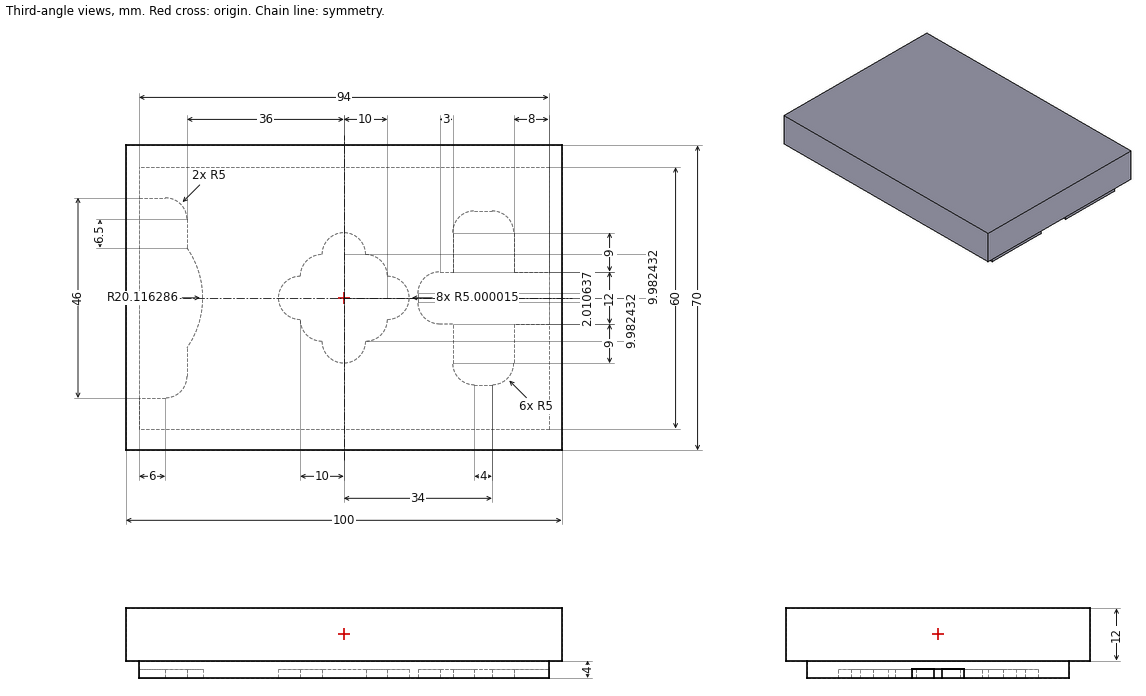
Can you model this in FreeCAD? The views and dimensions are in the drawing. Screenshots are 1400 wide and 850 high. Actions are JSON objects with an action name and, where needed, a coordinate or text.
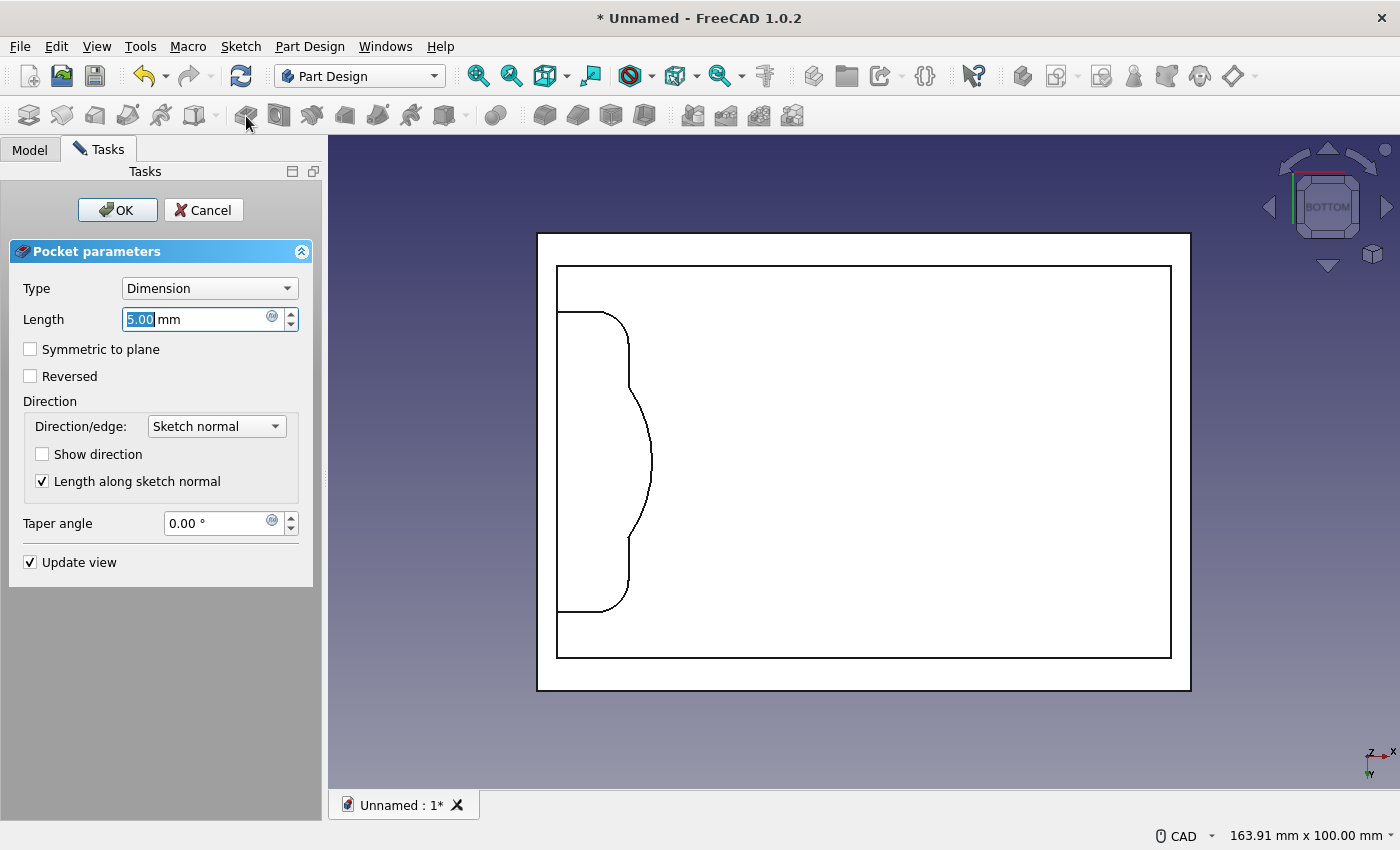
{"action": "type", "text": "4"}
{"action": "key", "text": "Tab"}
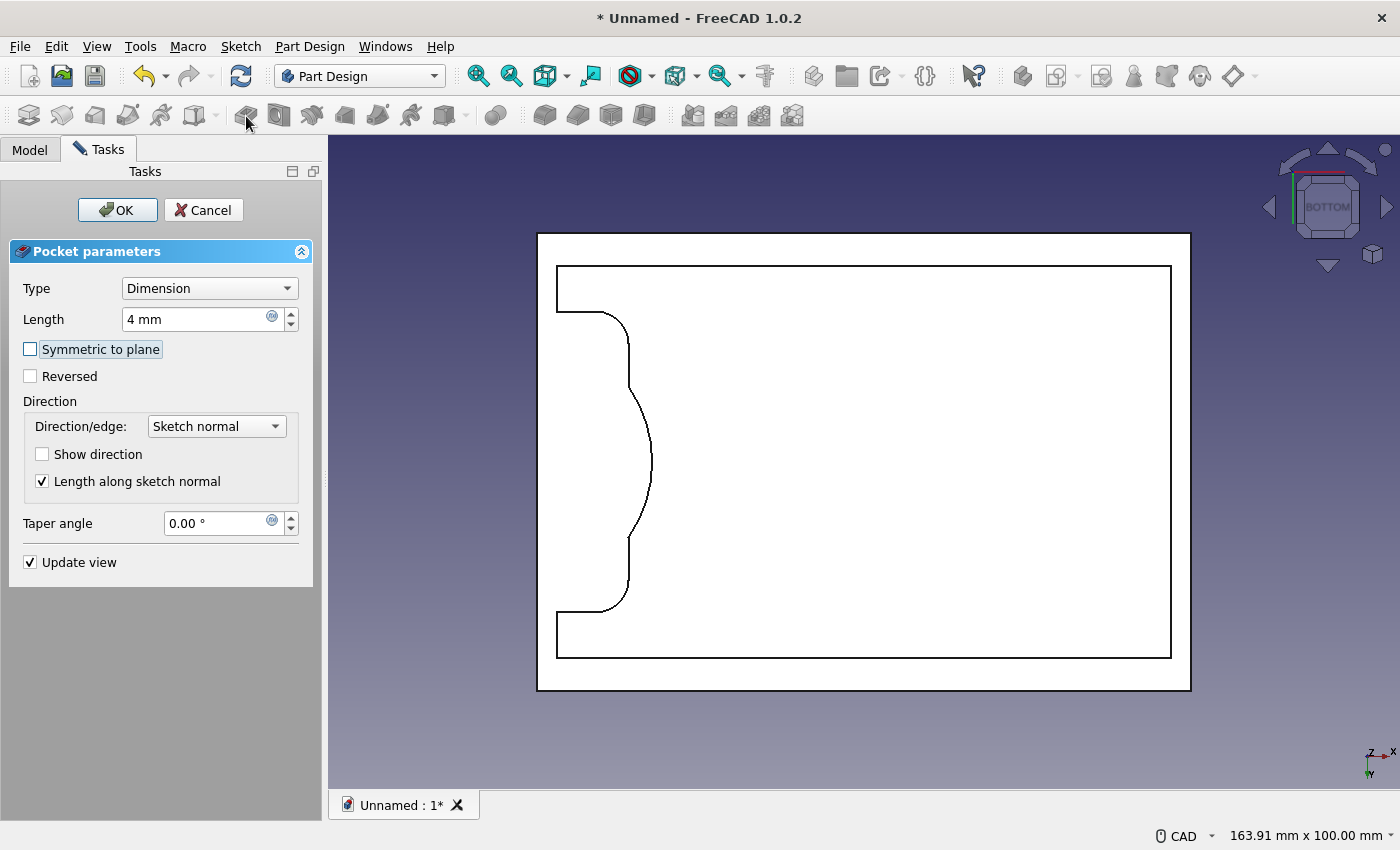
{"action": "left_click", "coordinate": [31, 349]}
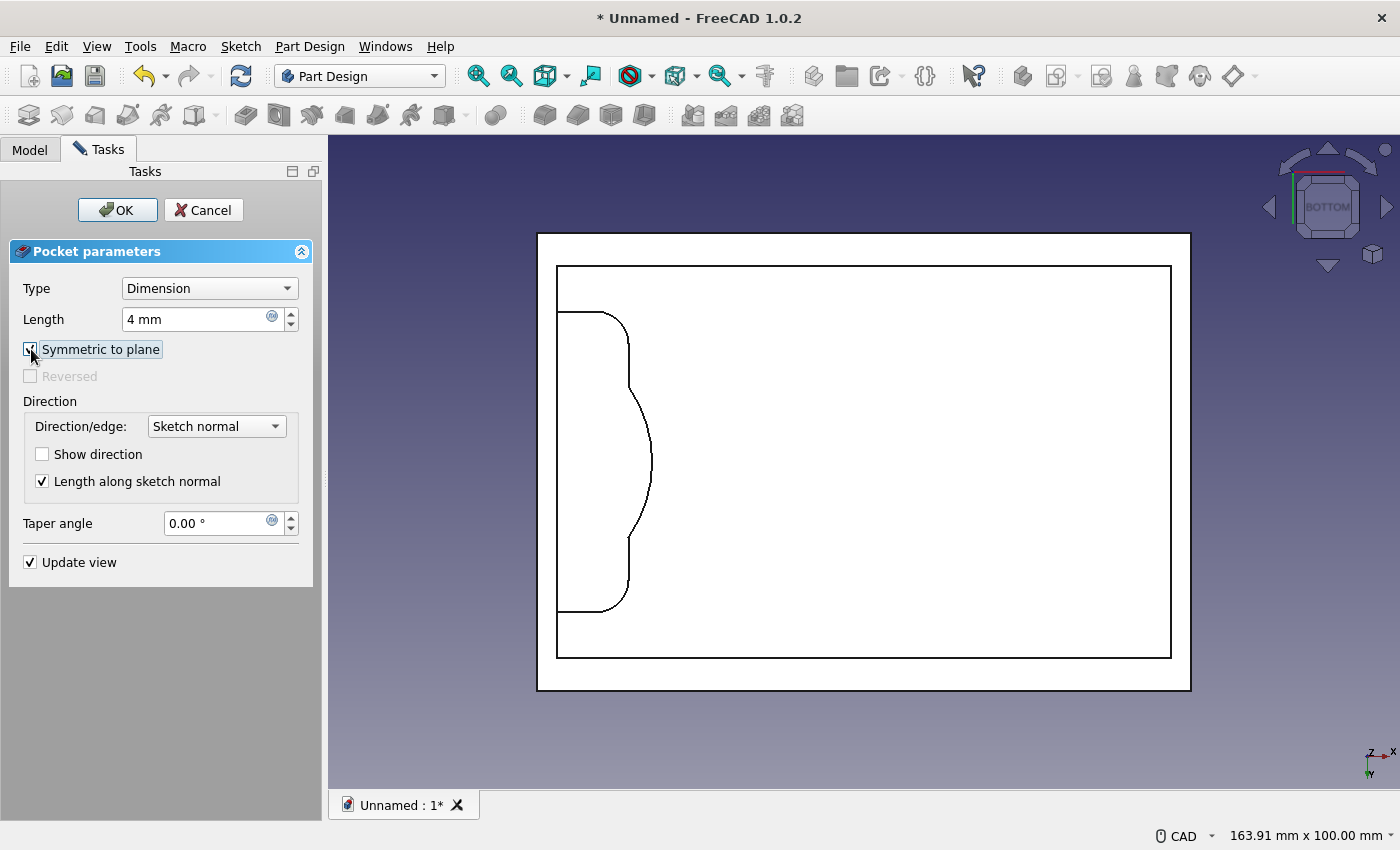
{"action": "left_click", "coordinate": [118, 210]}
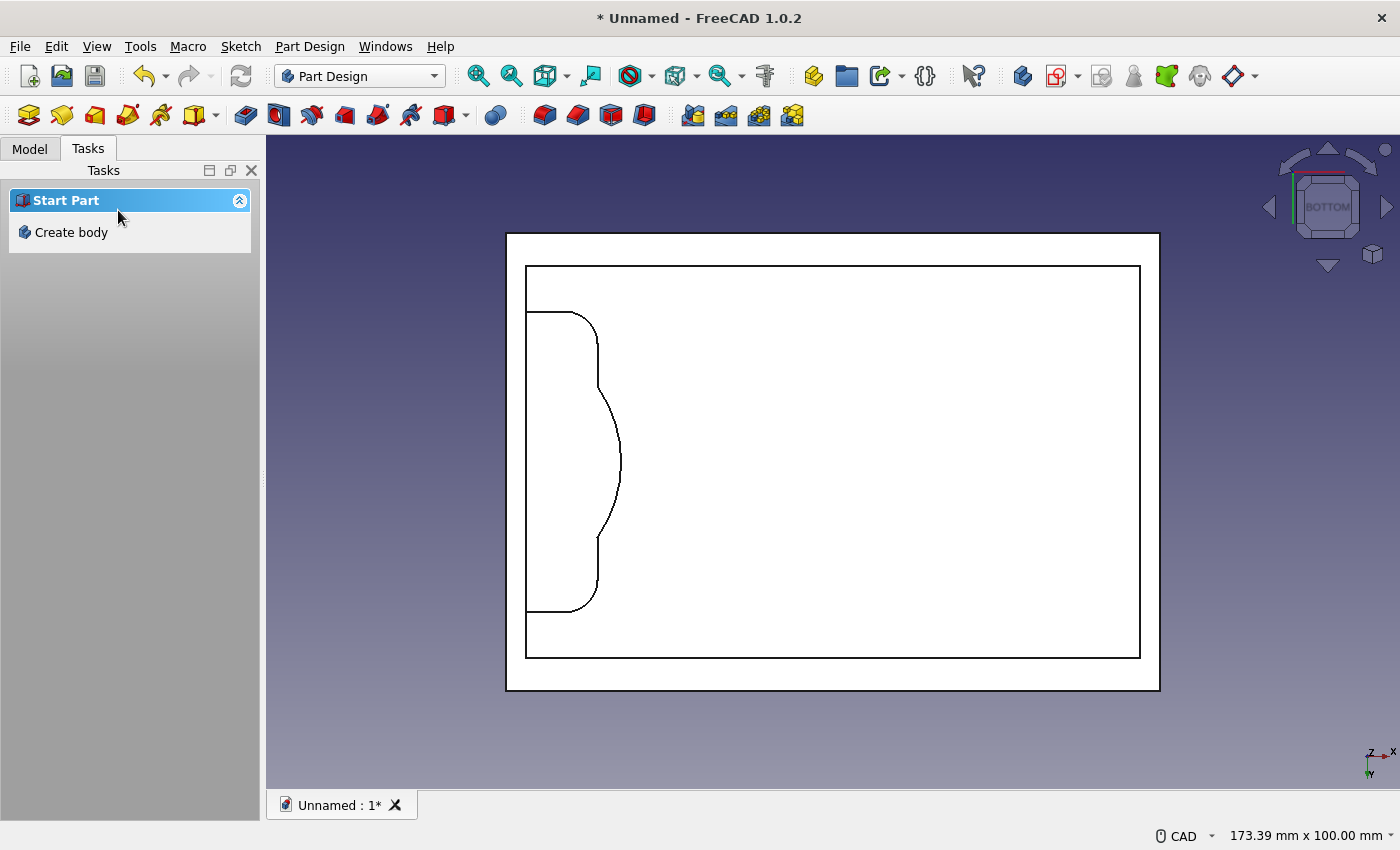
{"action": "left_click", "coordinate": [921, 461]}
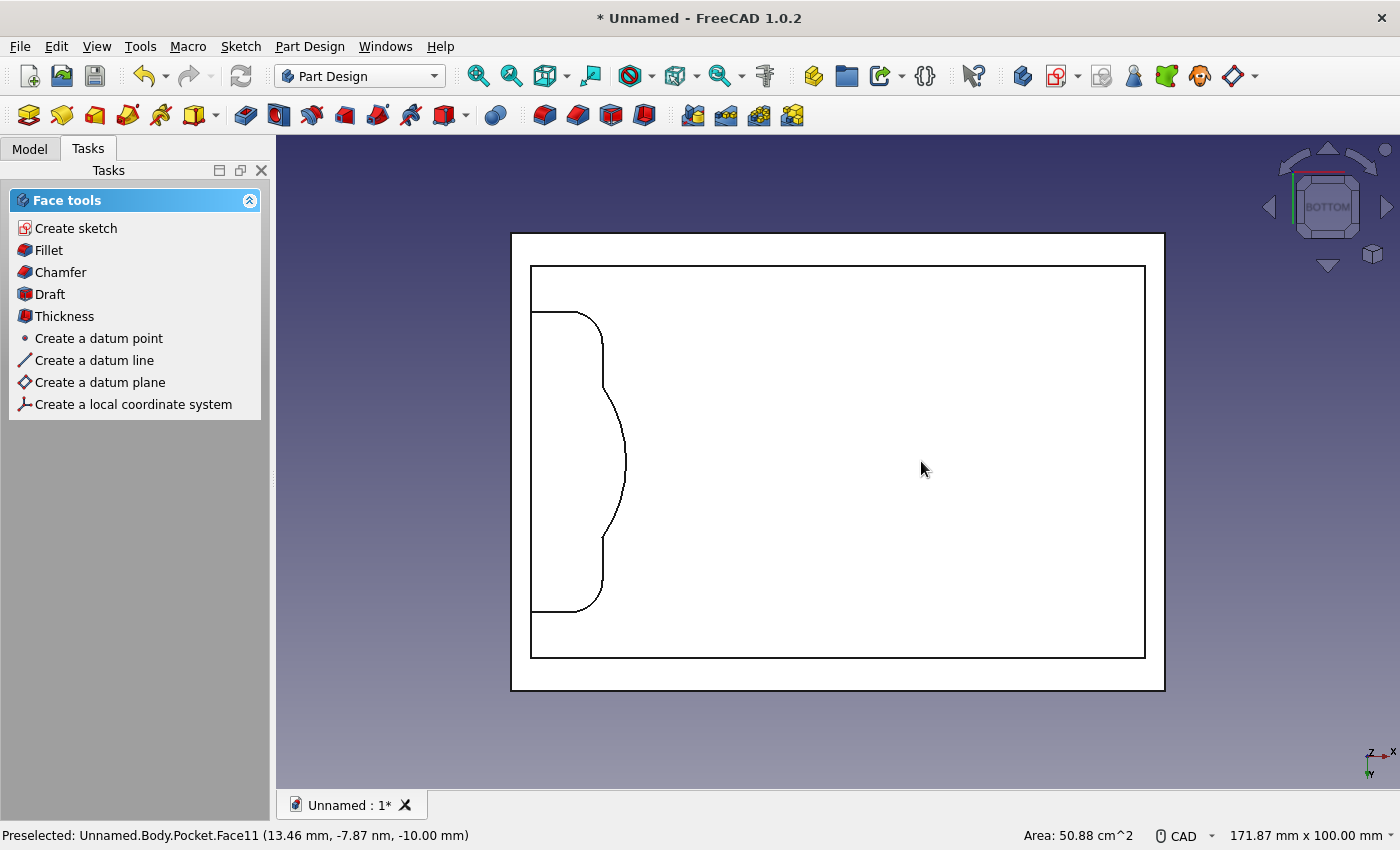
{"action": "left_click", "coordinate": [1056, 76]}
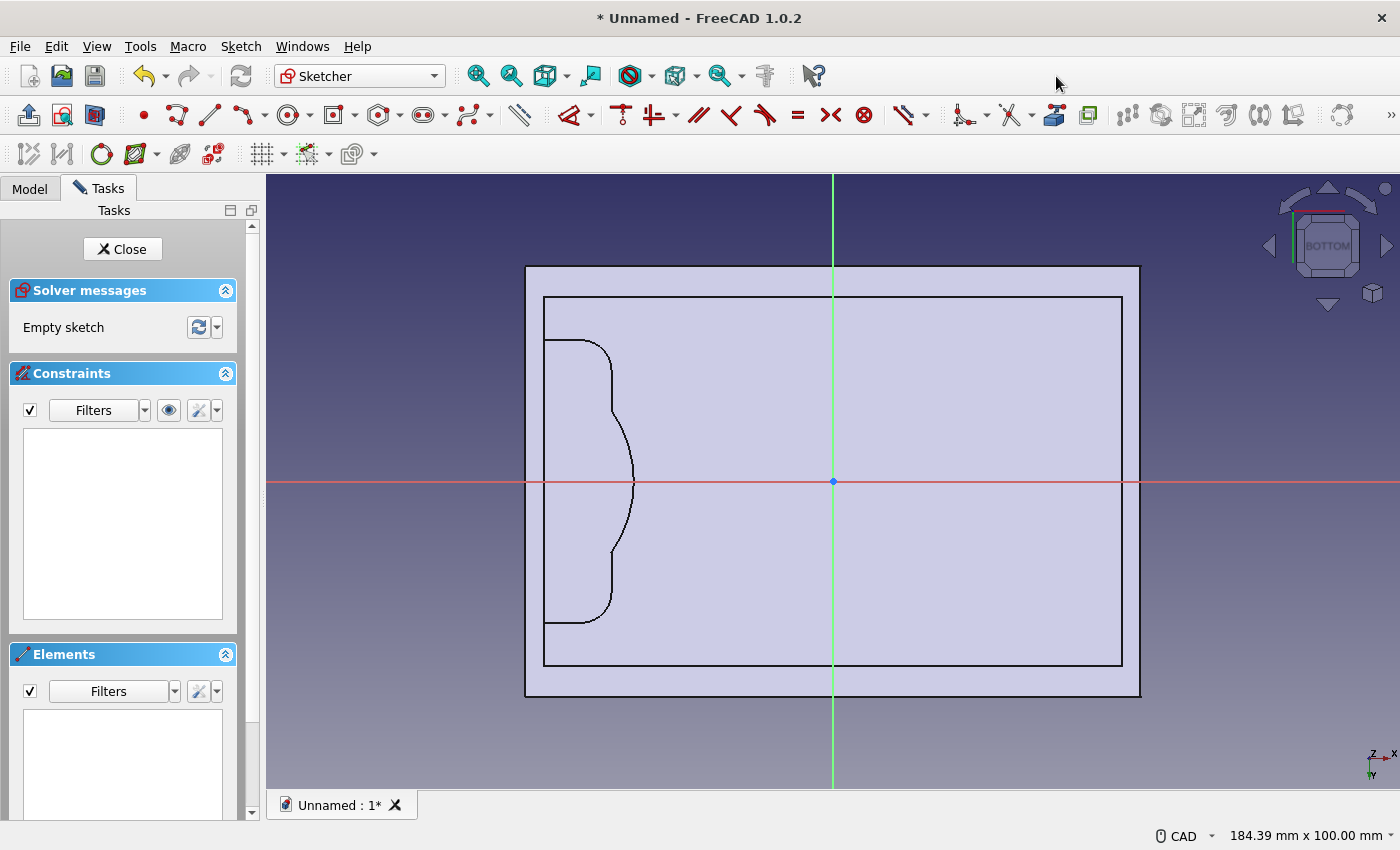
{"action": "scroll", "coordinate": [1235, 482], "scroll_direction": "up", "scroll_amount": 2}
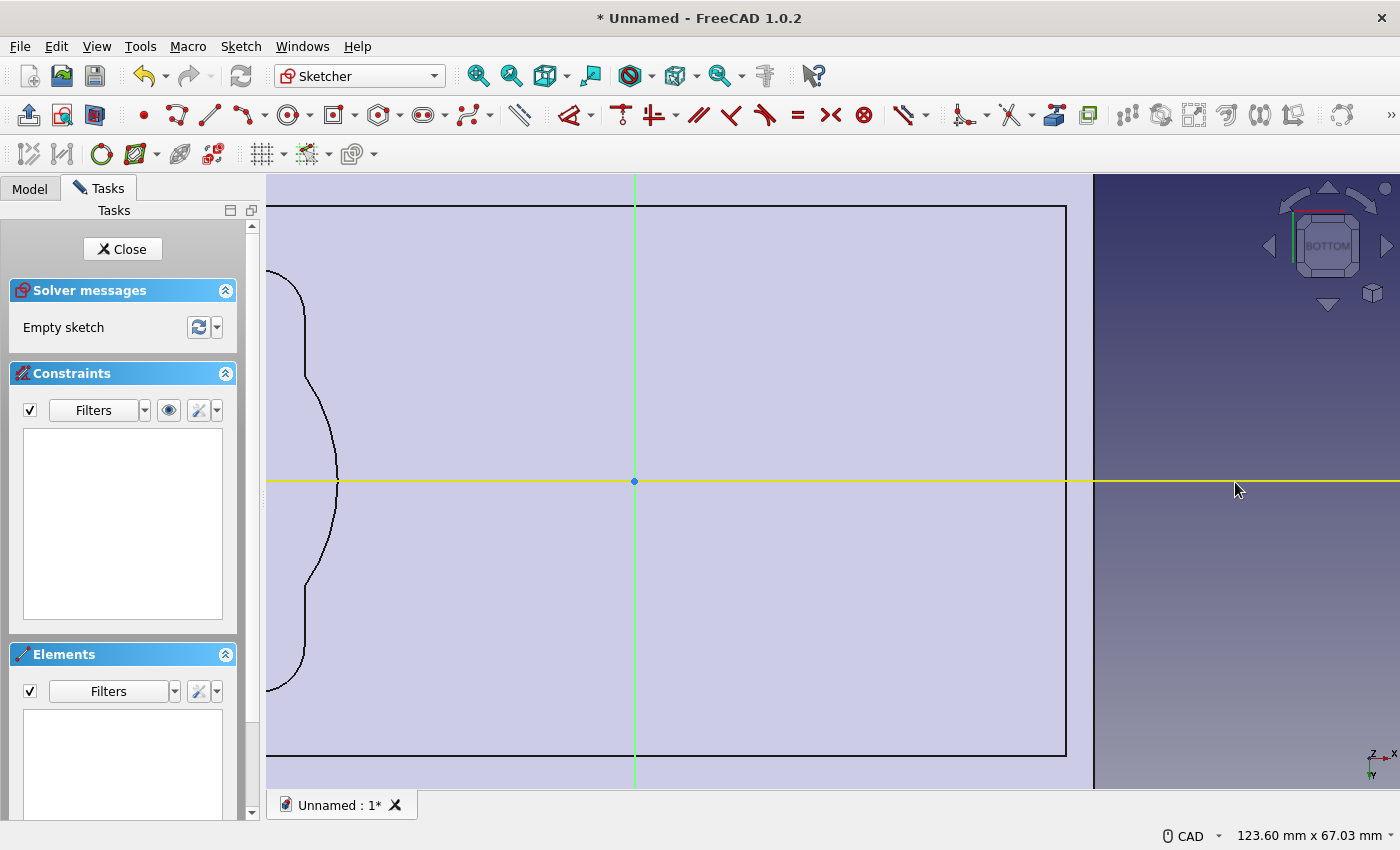
{"action": "left_click", "coordinate": [210, 116]}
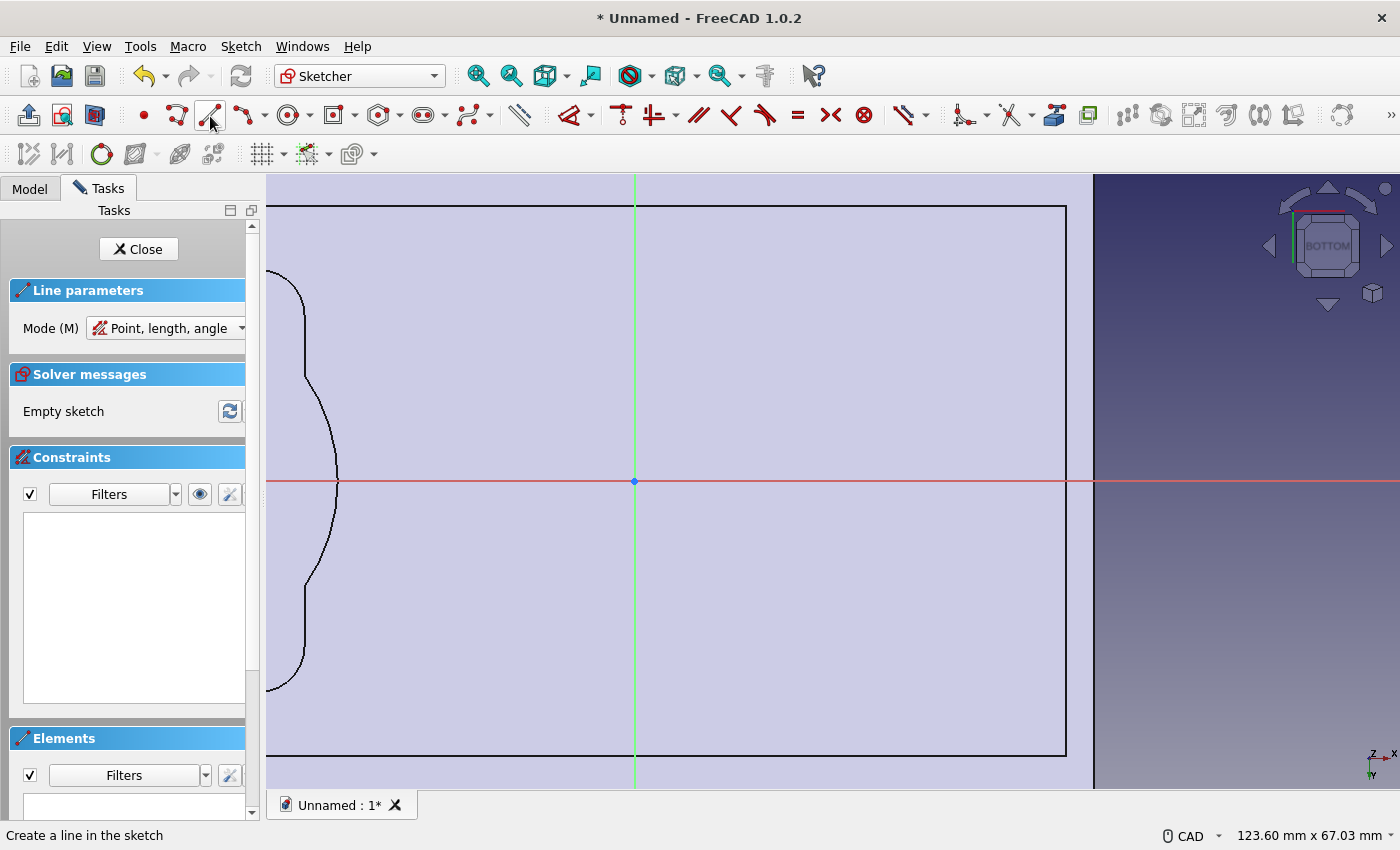
{"action": "left_click", "coordinate": [947, 298]}
{"action": "left_click", "coordinate": [910, 298]}